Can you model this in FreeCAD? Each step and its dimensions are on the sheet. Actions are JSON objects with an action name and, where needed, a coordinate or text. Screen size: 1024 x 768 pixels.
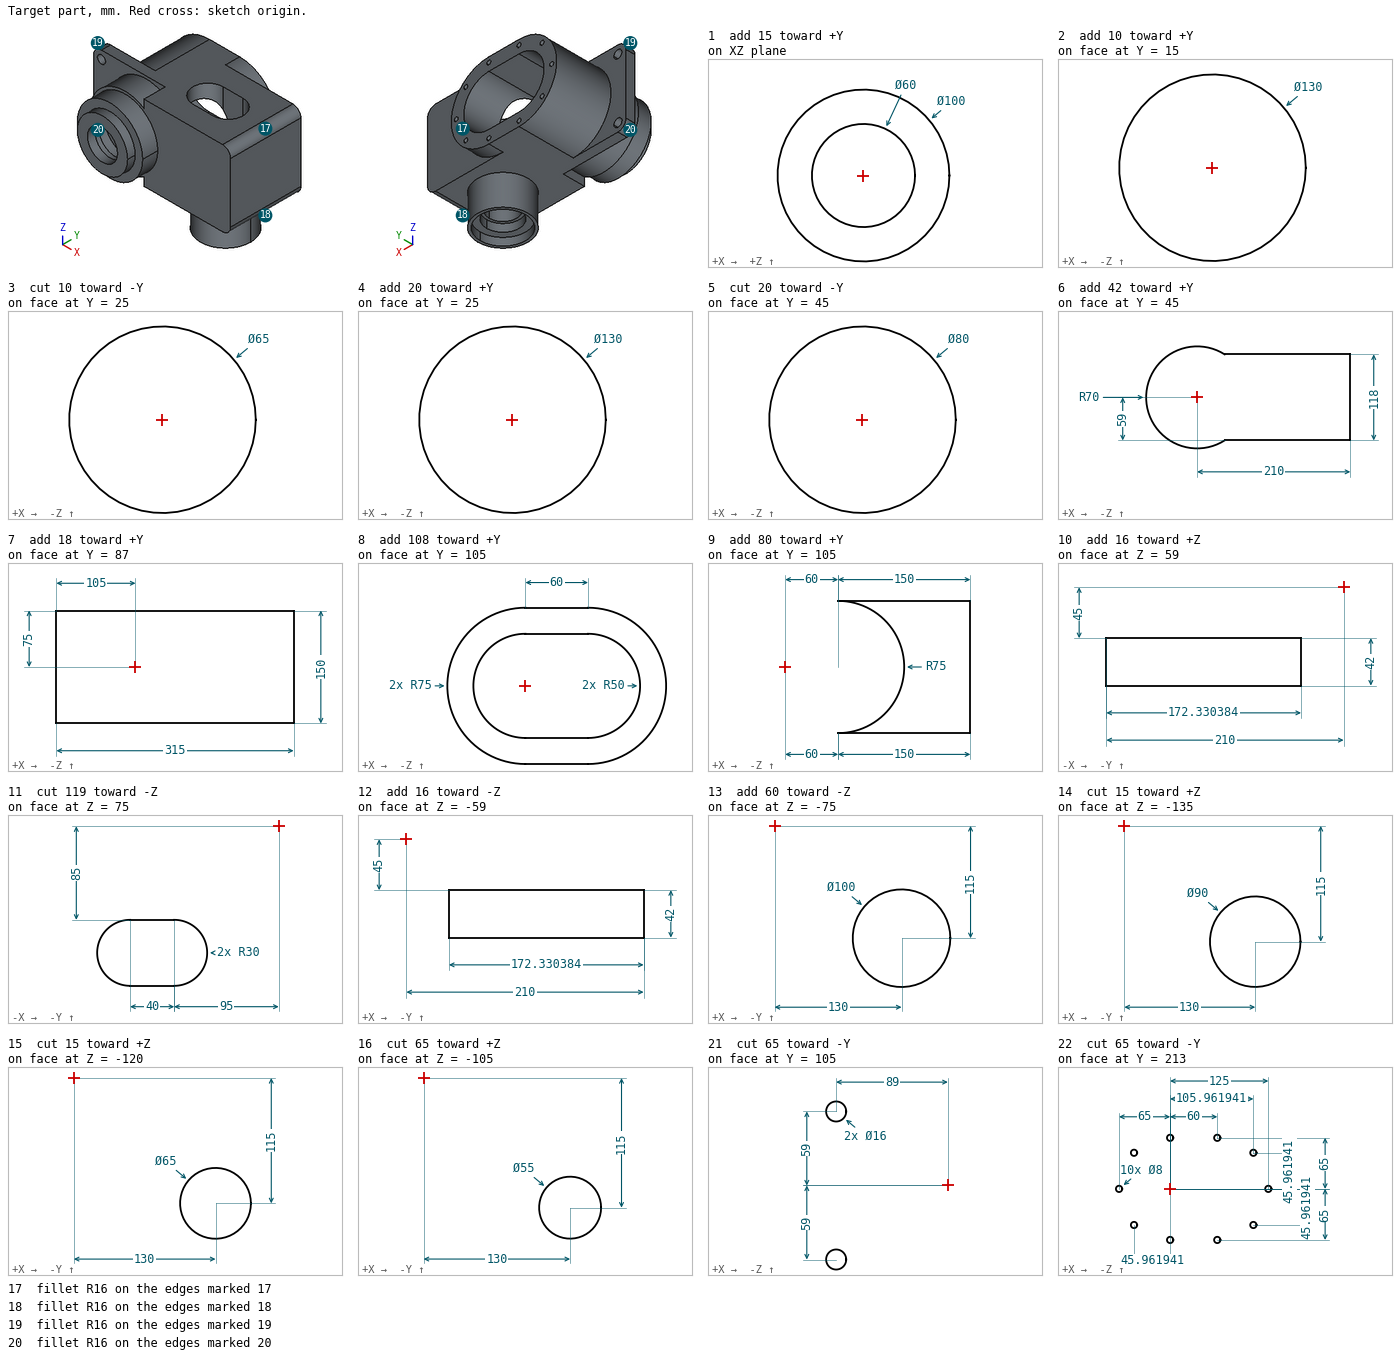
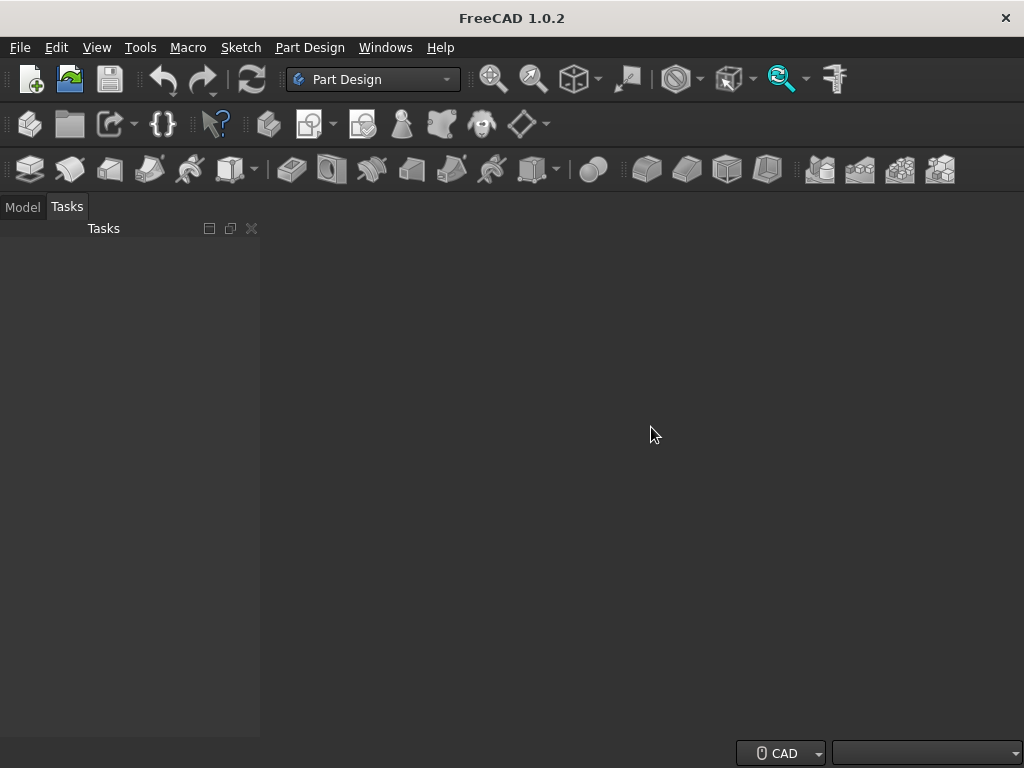
{"action": "left_click", "coordinate": [30, 80]}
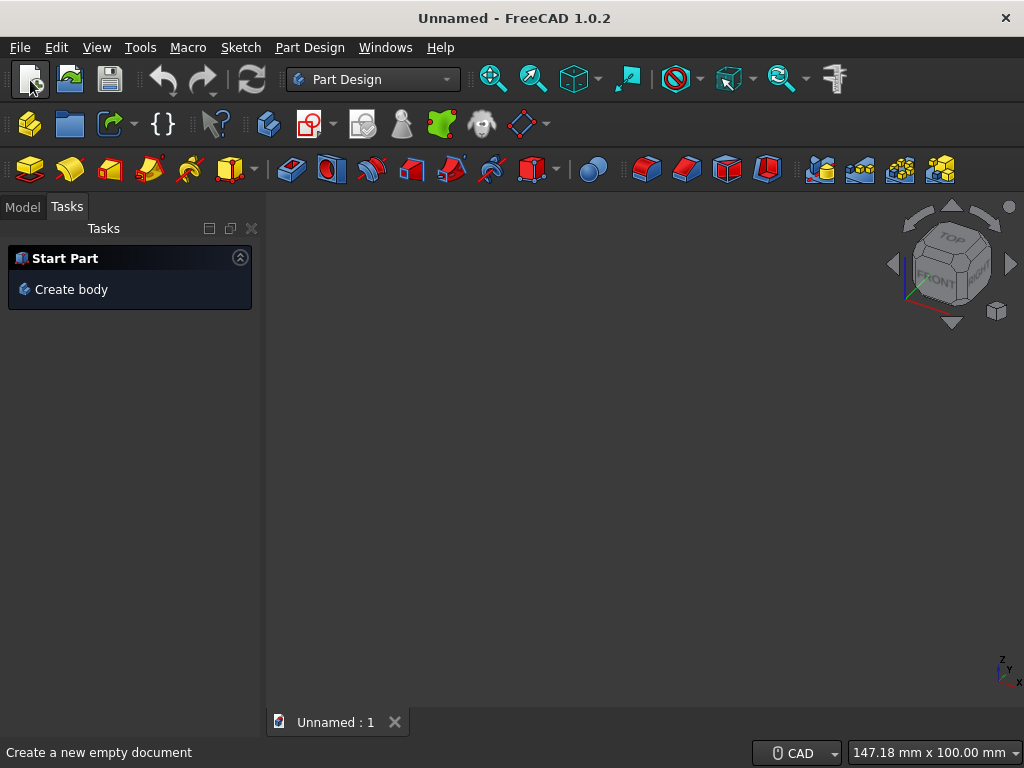
{"action": "left_click", "coordinate": [310, 124]}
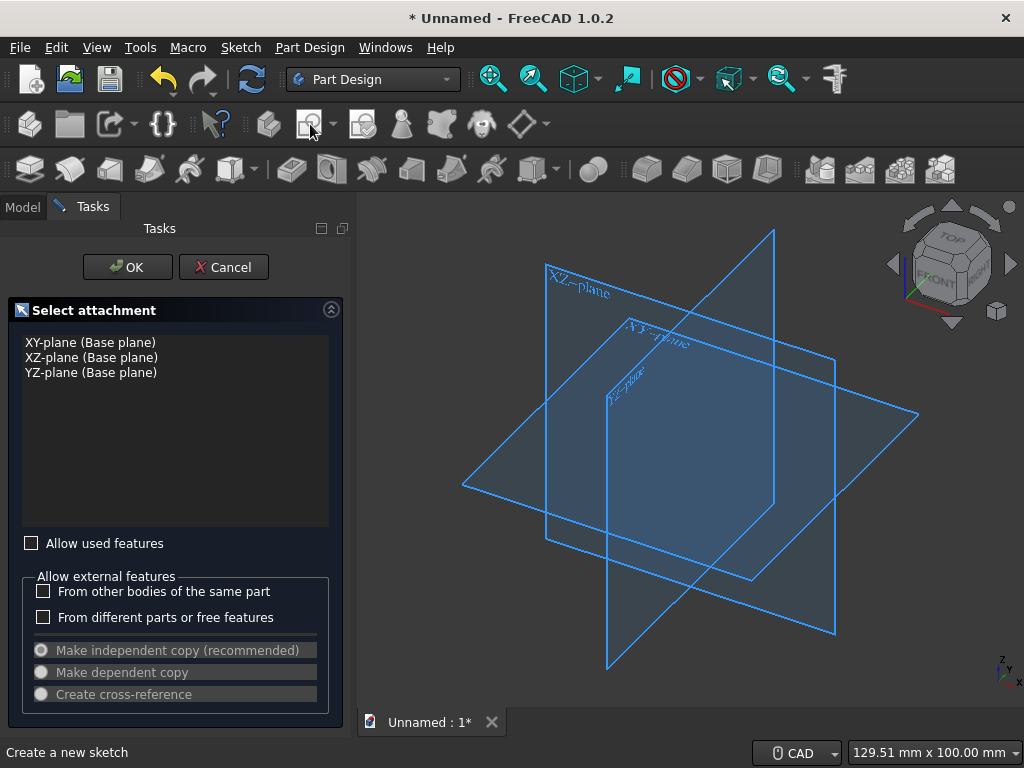
{"action": "left_click", "coordinate": [82, 358]}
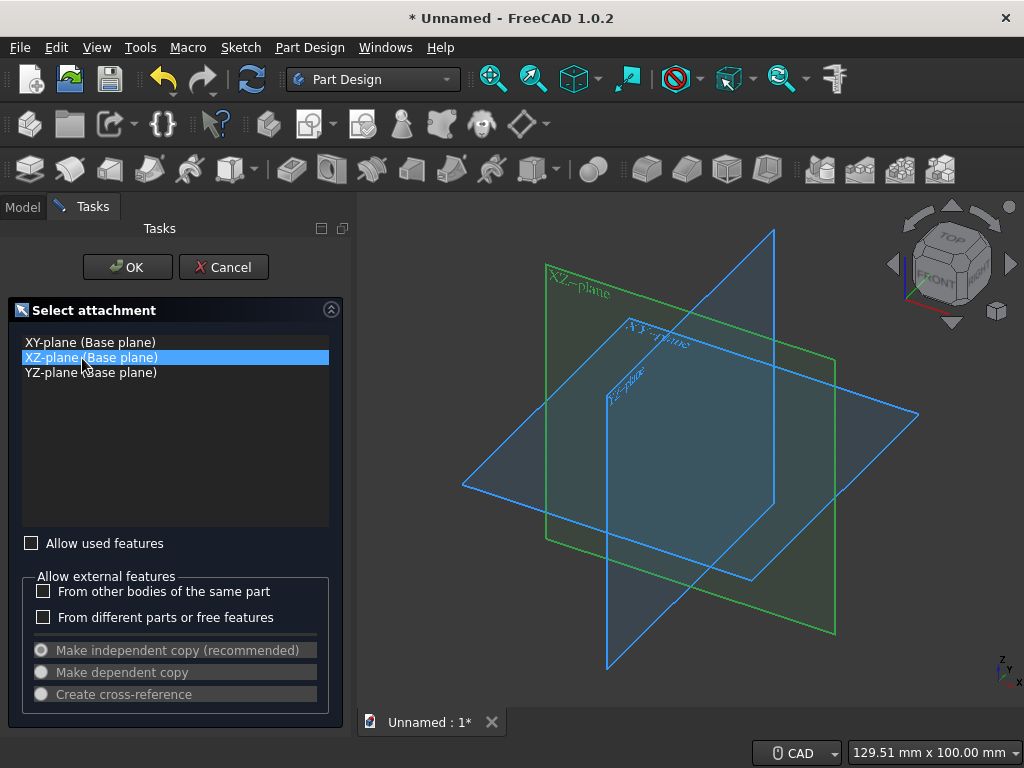
{"action": "left_click", "coordinate": [128, 267]}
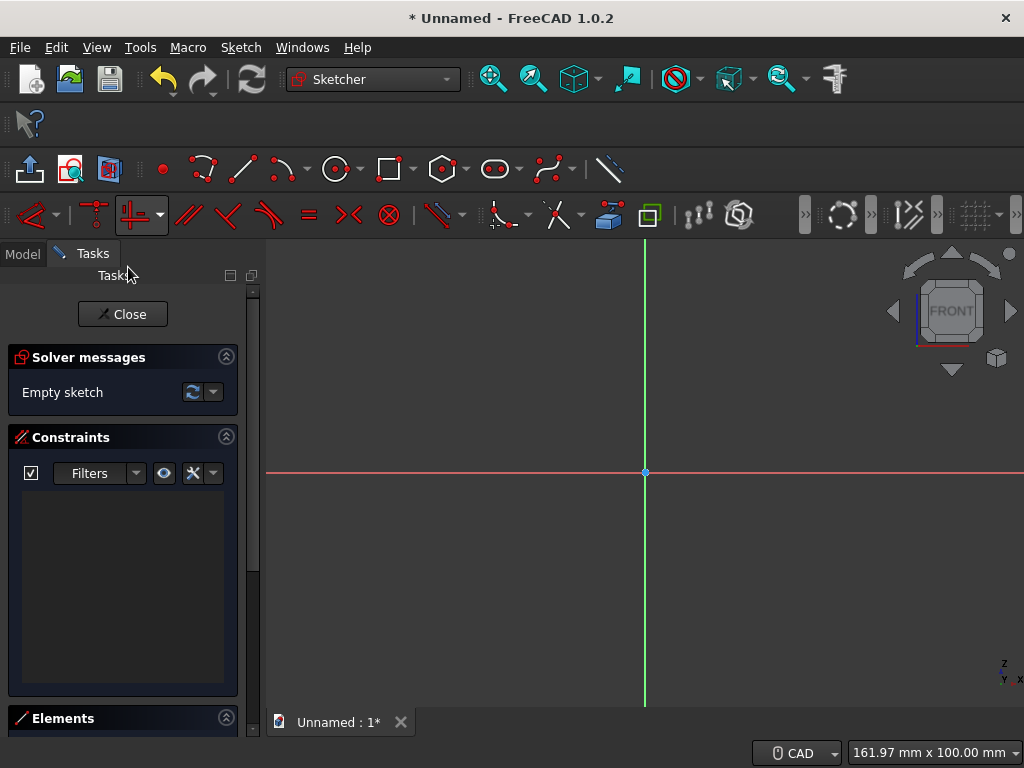
{"action": "scroll", "coordinate": [437, 473], "scroll_direction": "down", "scroll_amount": 2}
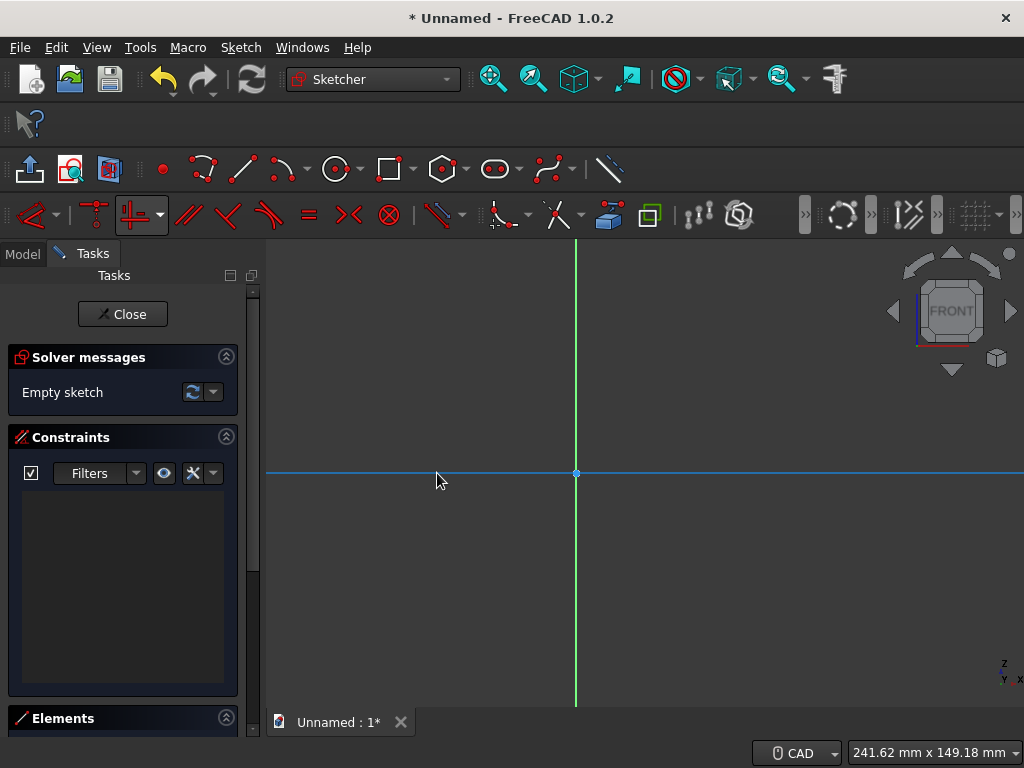
{"action": "left_click", "coordinate": [336, 170]}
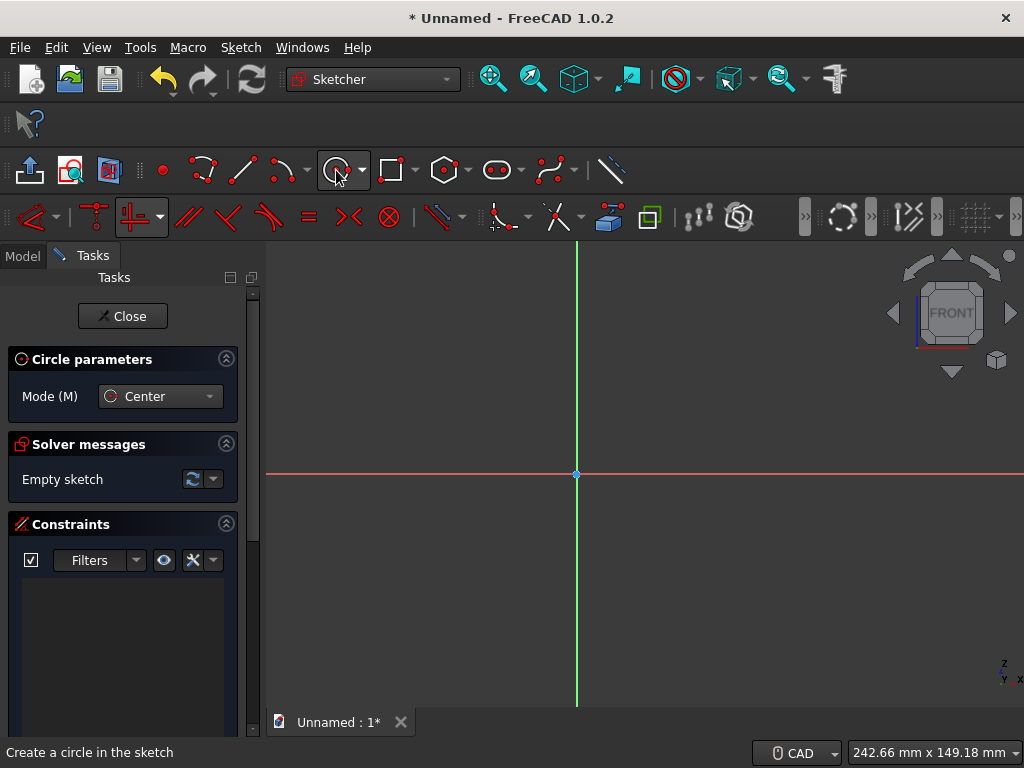
{"action": "left_click", "coordinate": [577, 474]}
{"action": "mouse_move", "coordinate": [687, 364]}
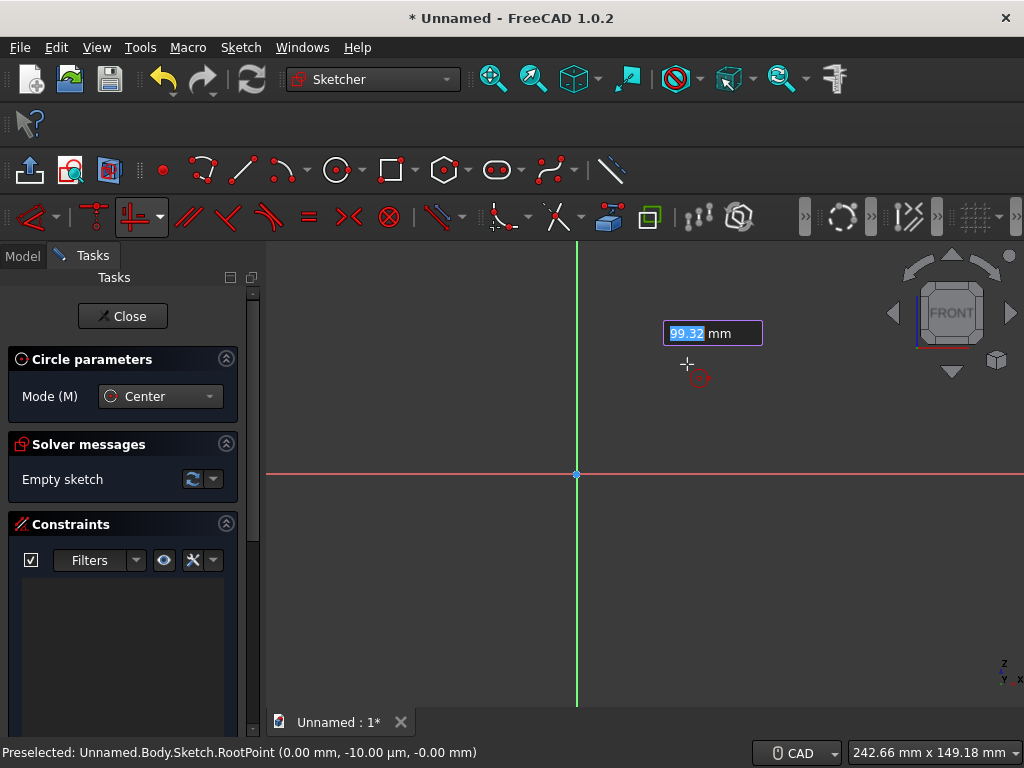
{"action": "type", "text": "100"}
{"action": "key", "text": "Return"}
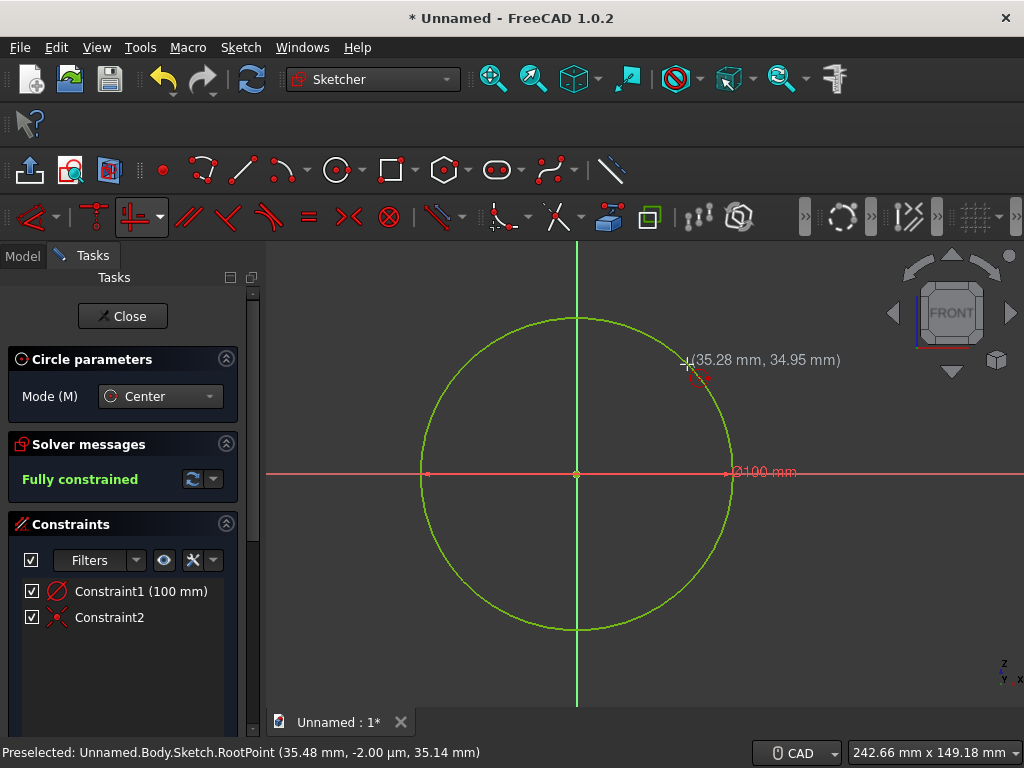
{"action": "left_click", "coordinate": [577, 474]}
{"action": "mouse_move", "coordinate": [643, 408]}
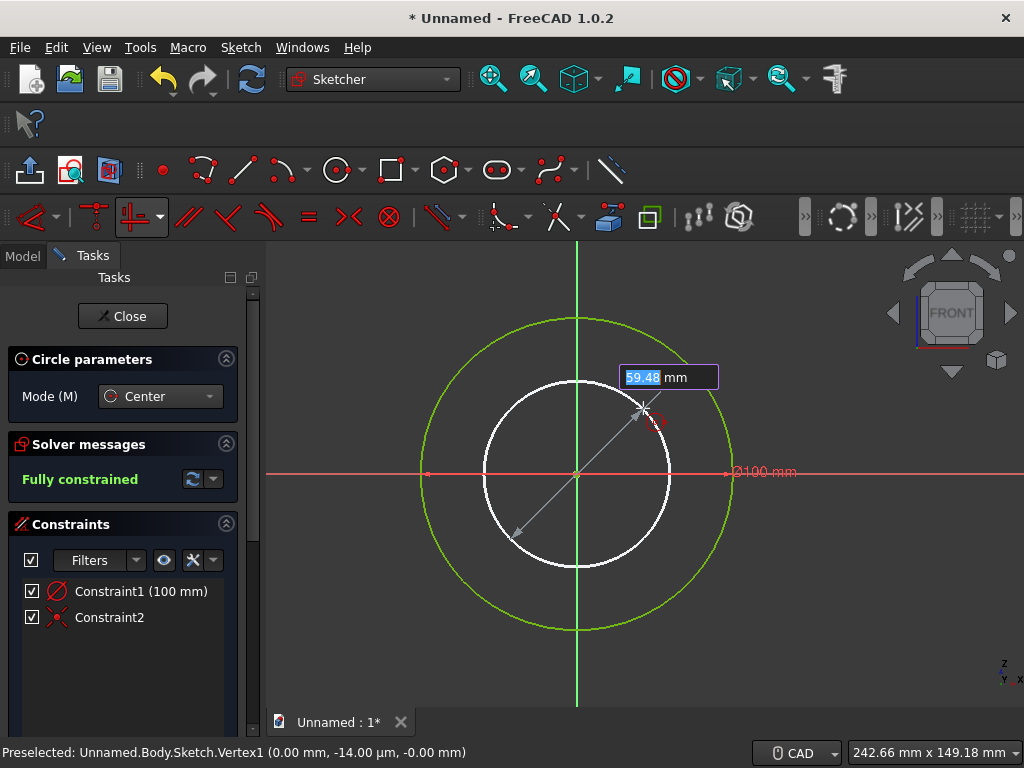
{"action": "type", "text": "60"}
{"action": "key", "text": "Return"}
{"action": "key", "text": "Escape"}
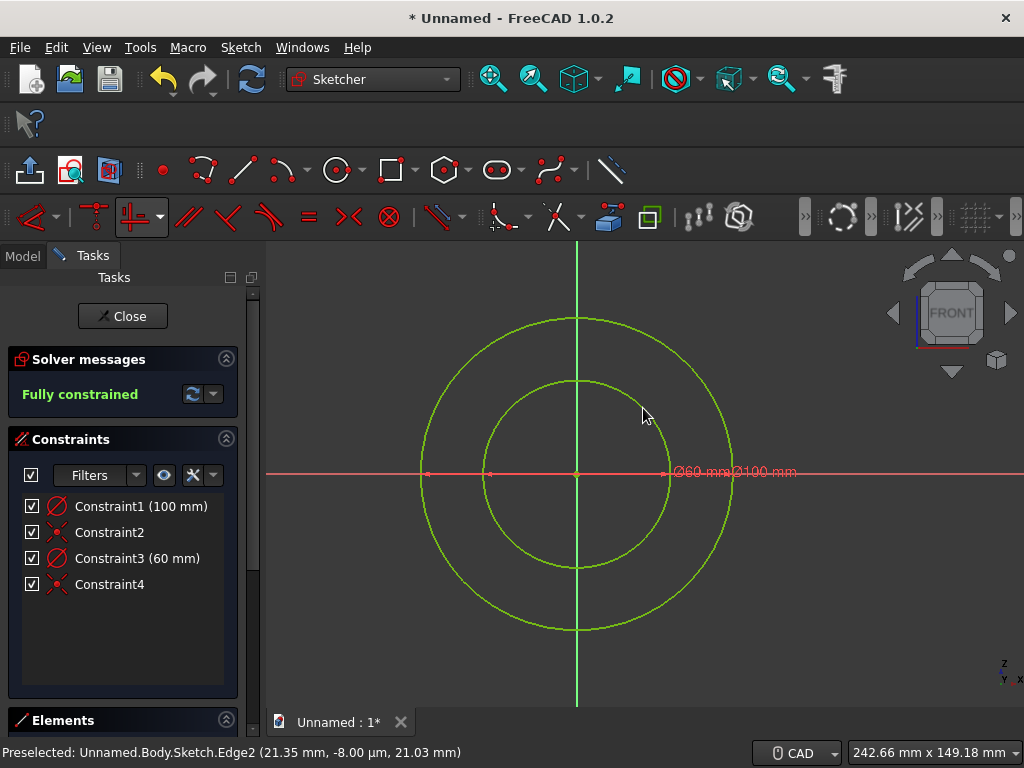
{"action": "left_click", "coordinate": [123, 316]}